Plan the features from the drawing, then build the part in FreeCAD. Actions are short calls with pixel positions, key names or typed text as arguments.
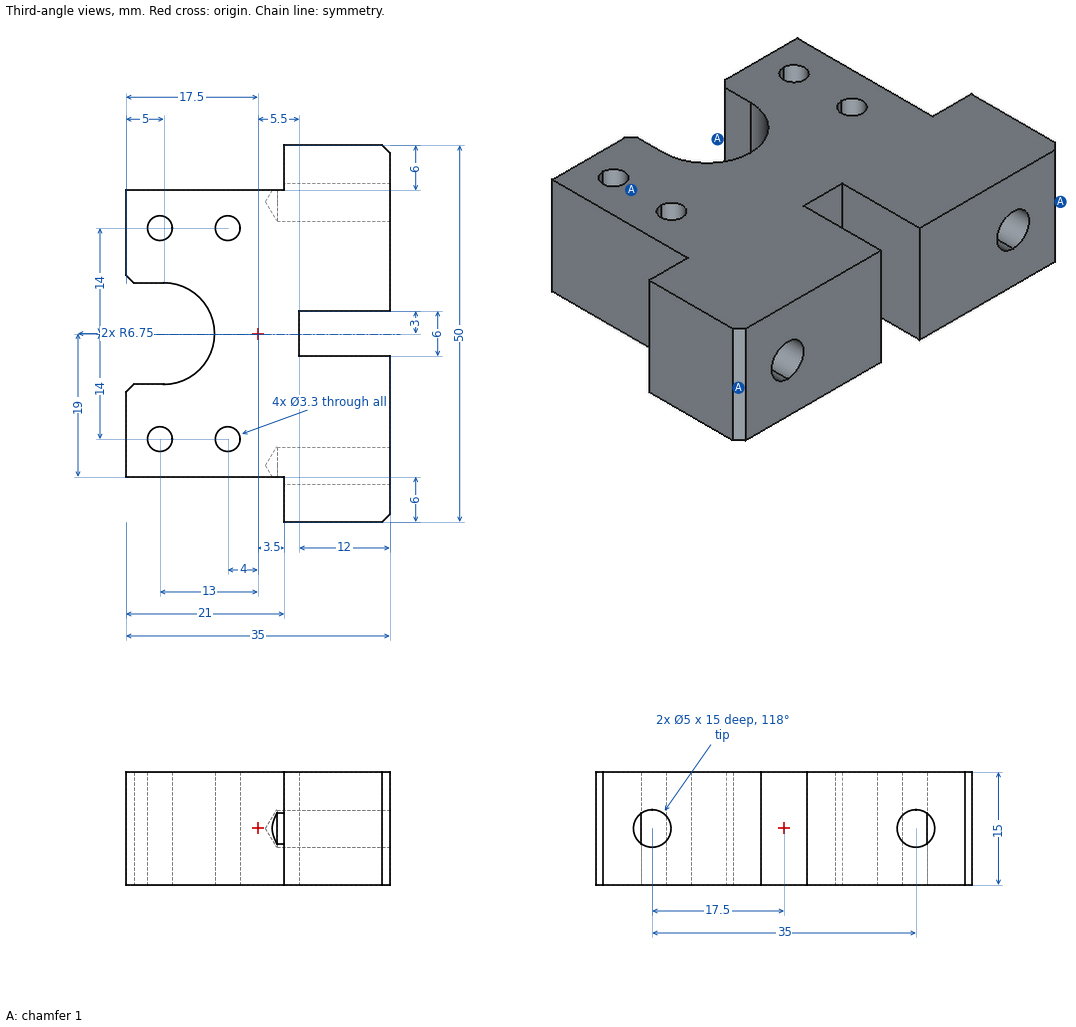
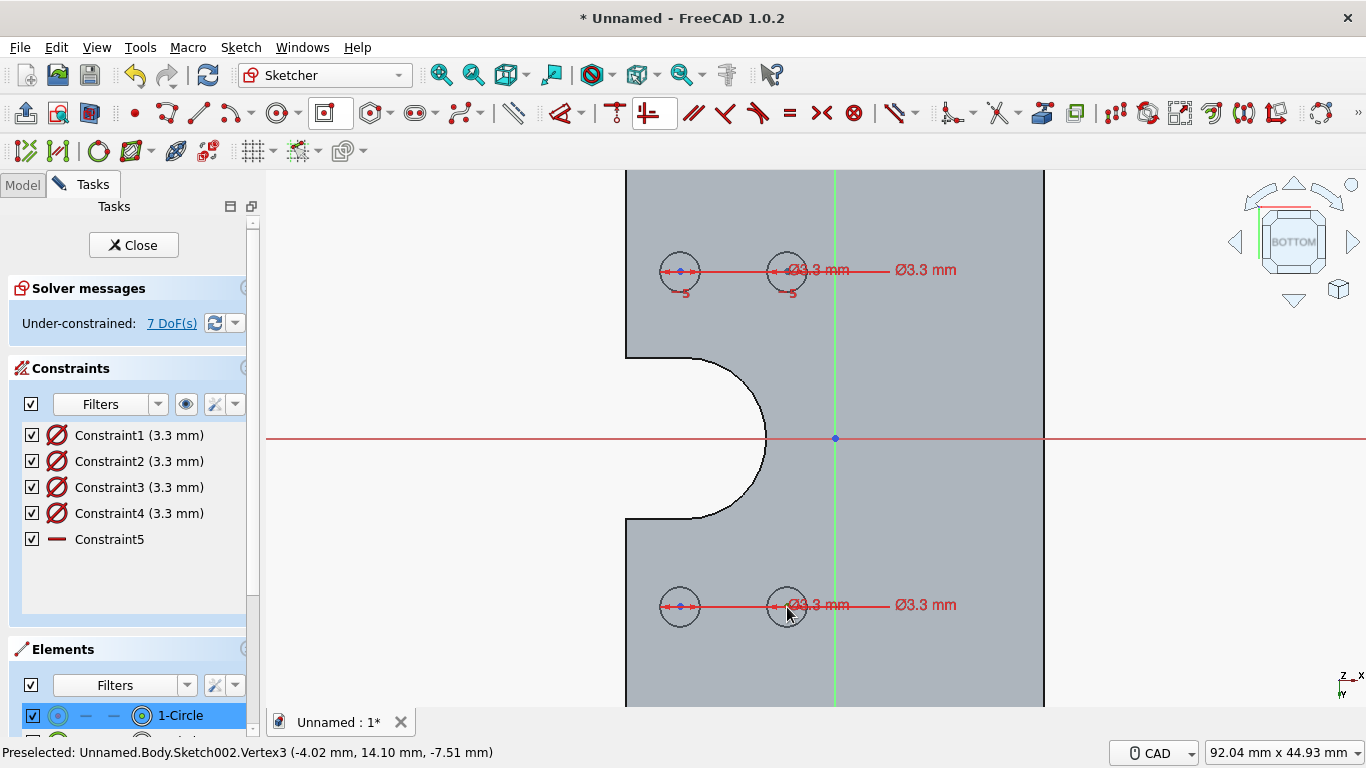
key(v)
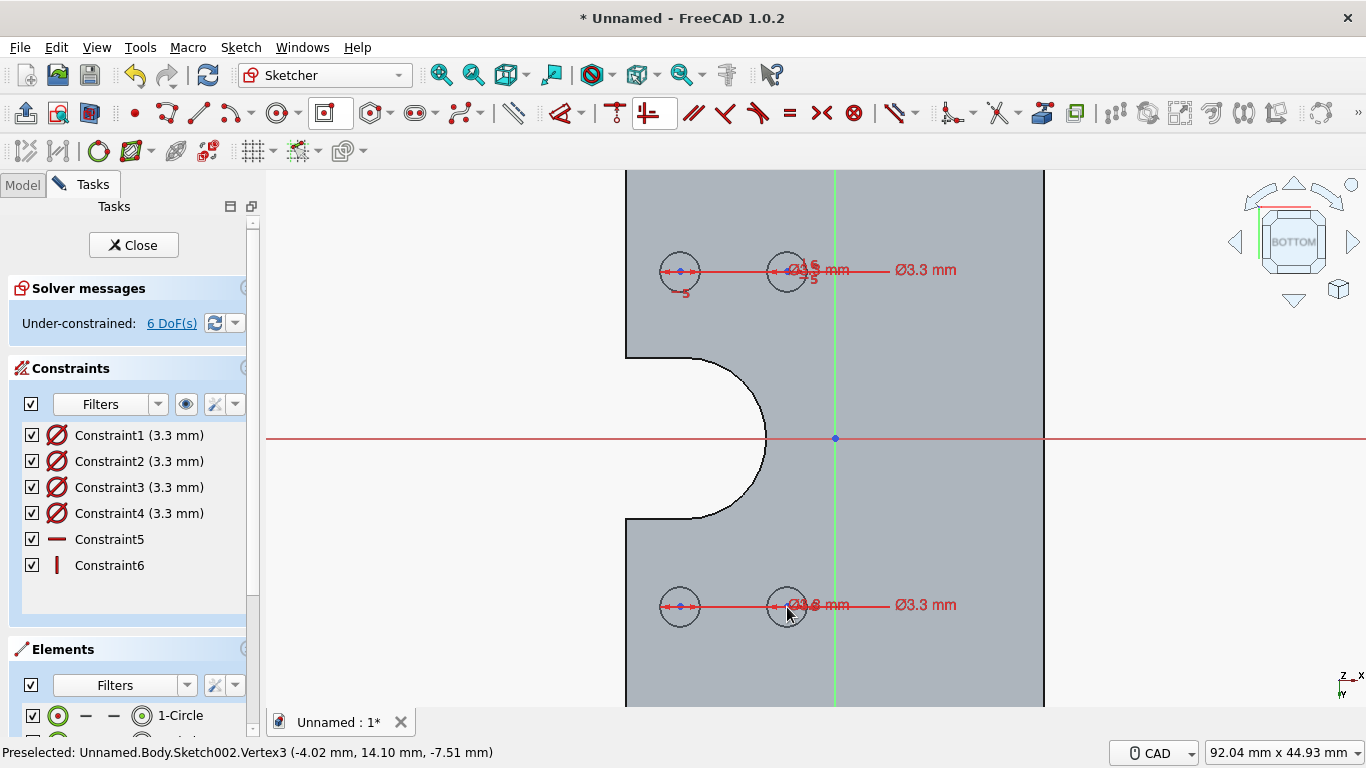
click(680, 272)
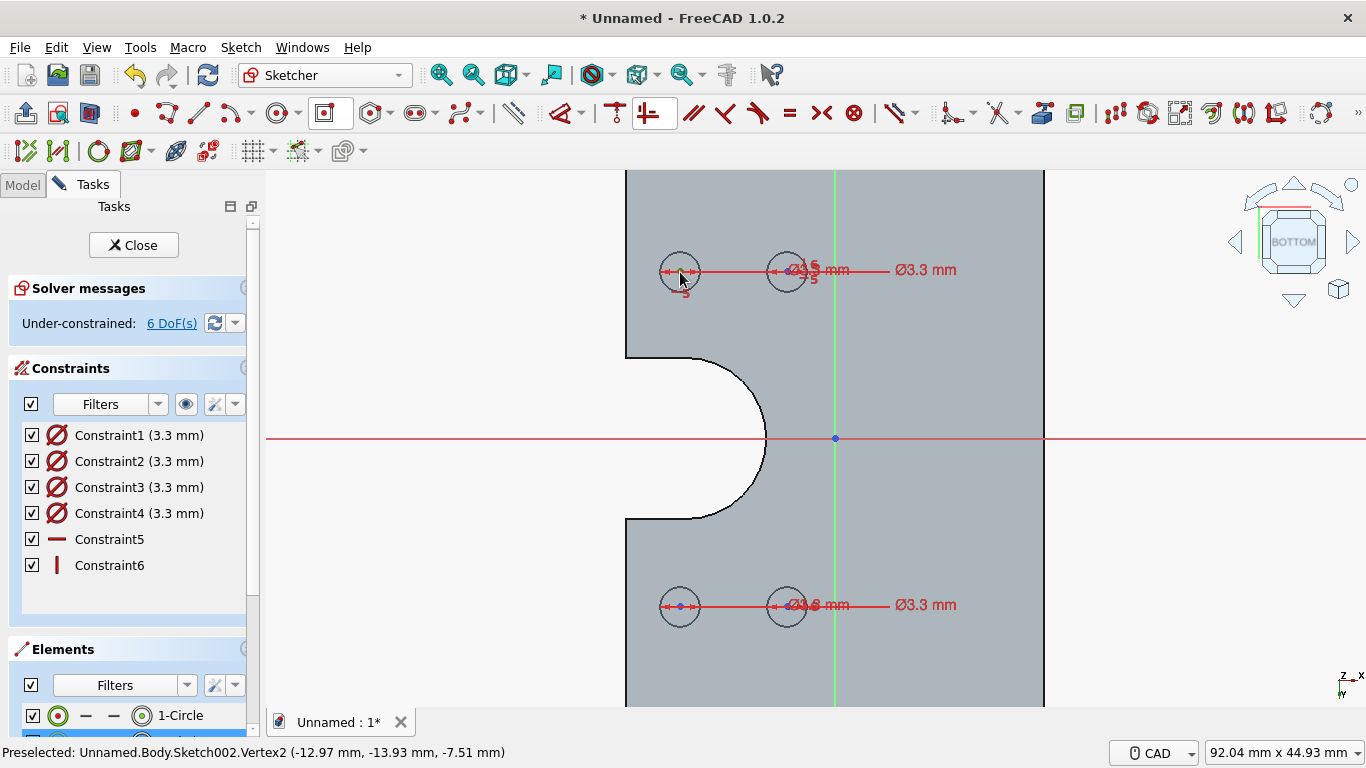
click(680, 607)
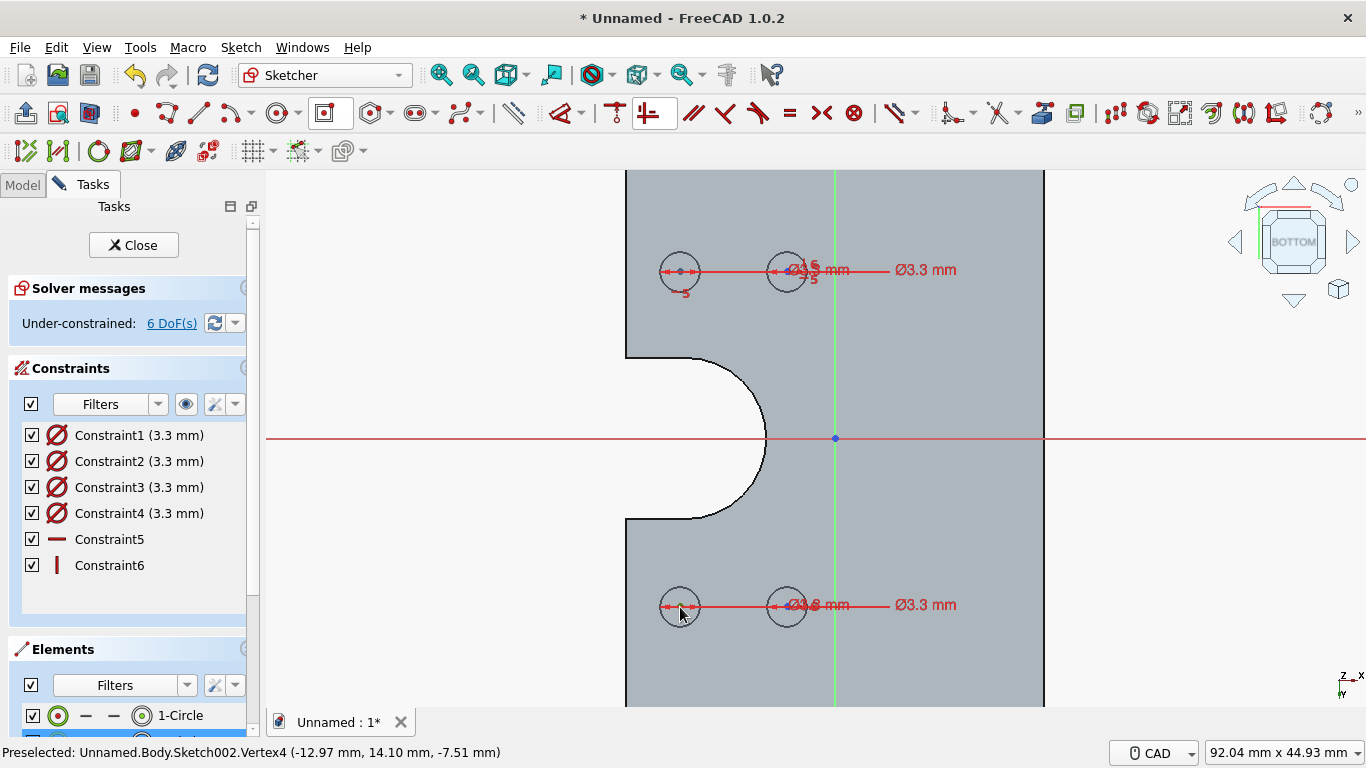
click(672, 114)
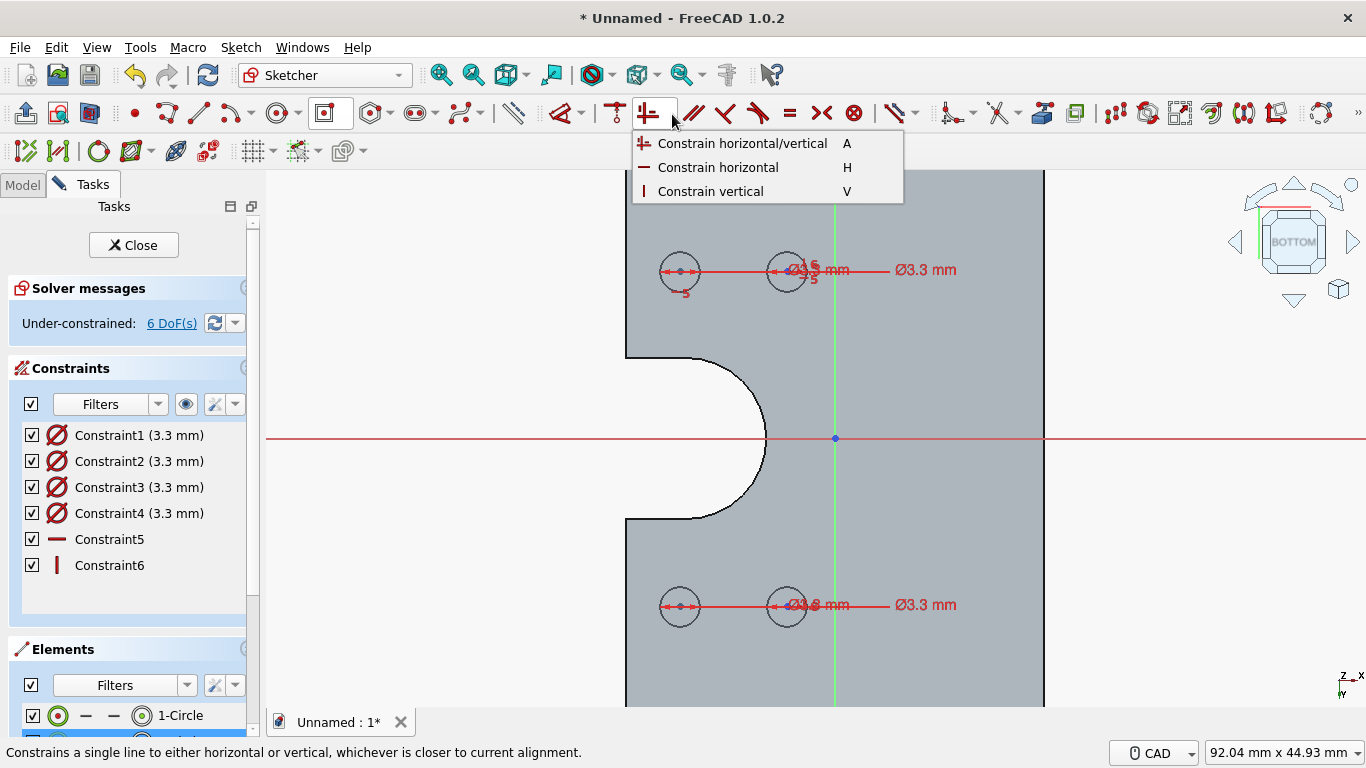
click(768, 191)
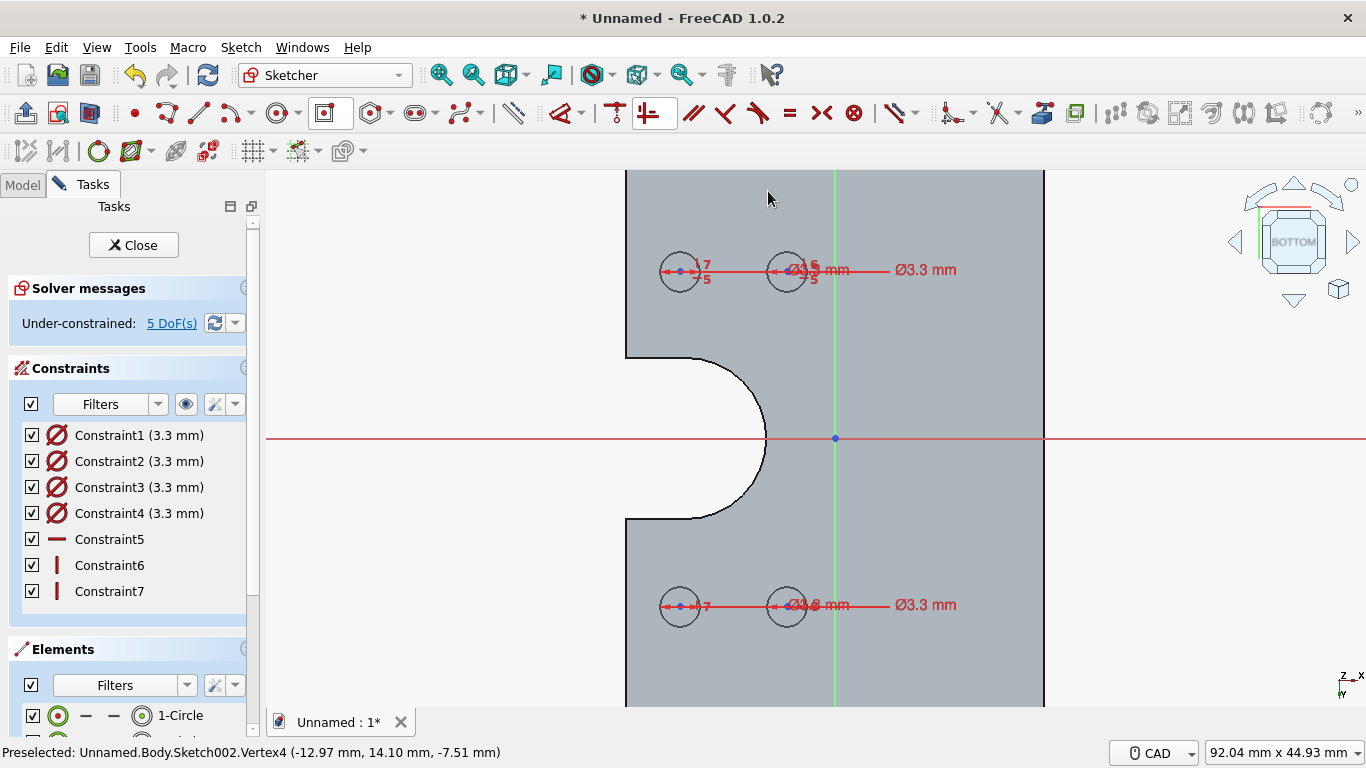
click(787, 607)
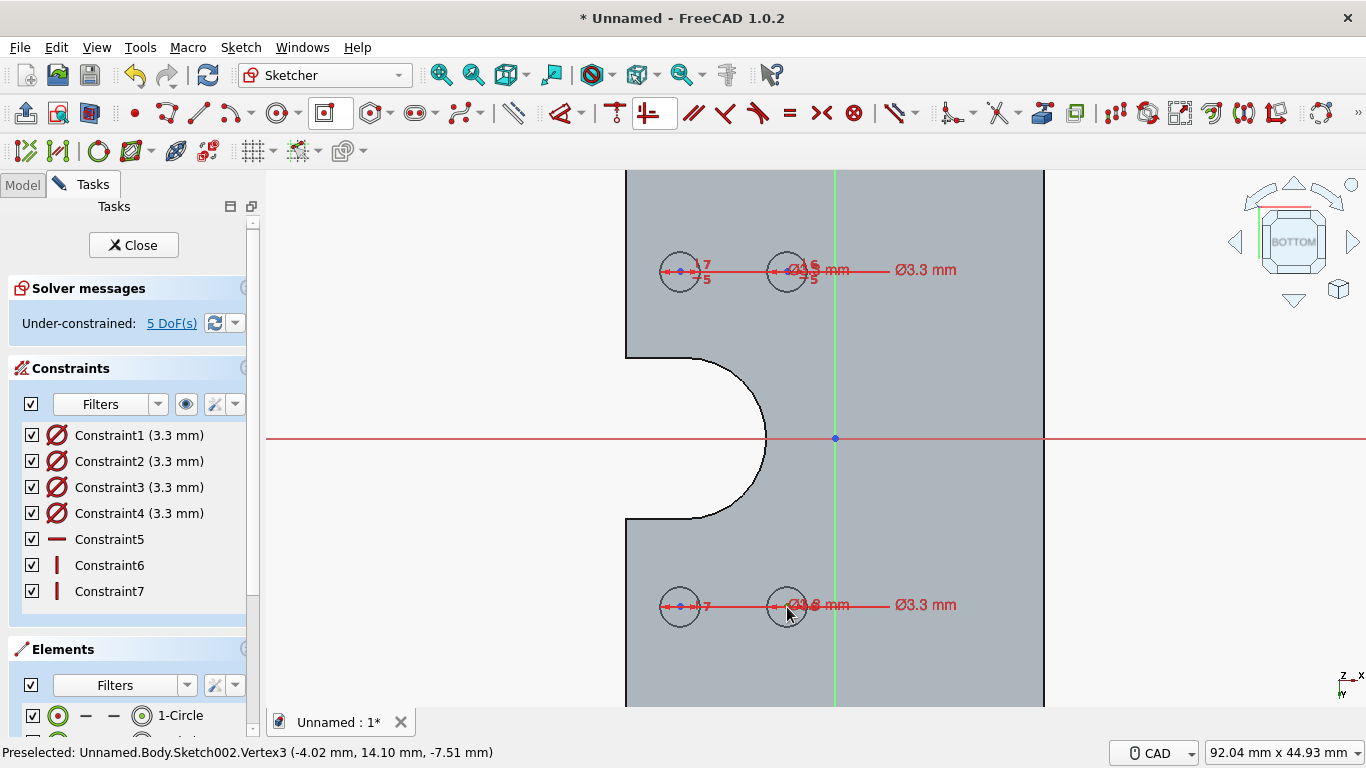
click(680, 607)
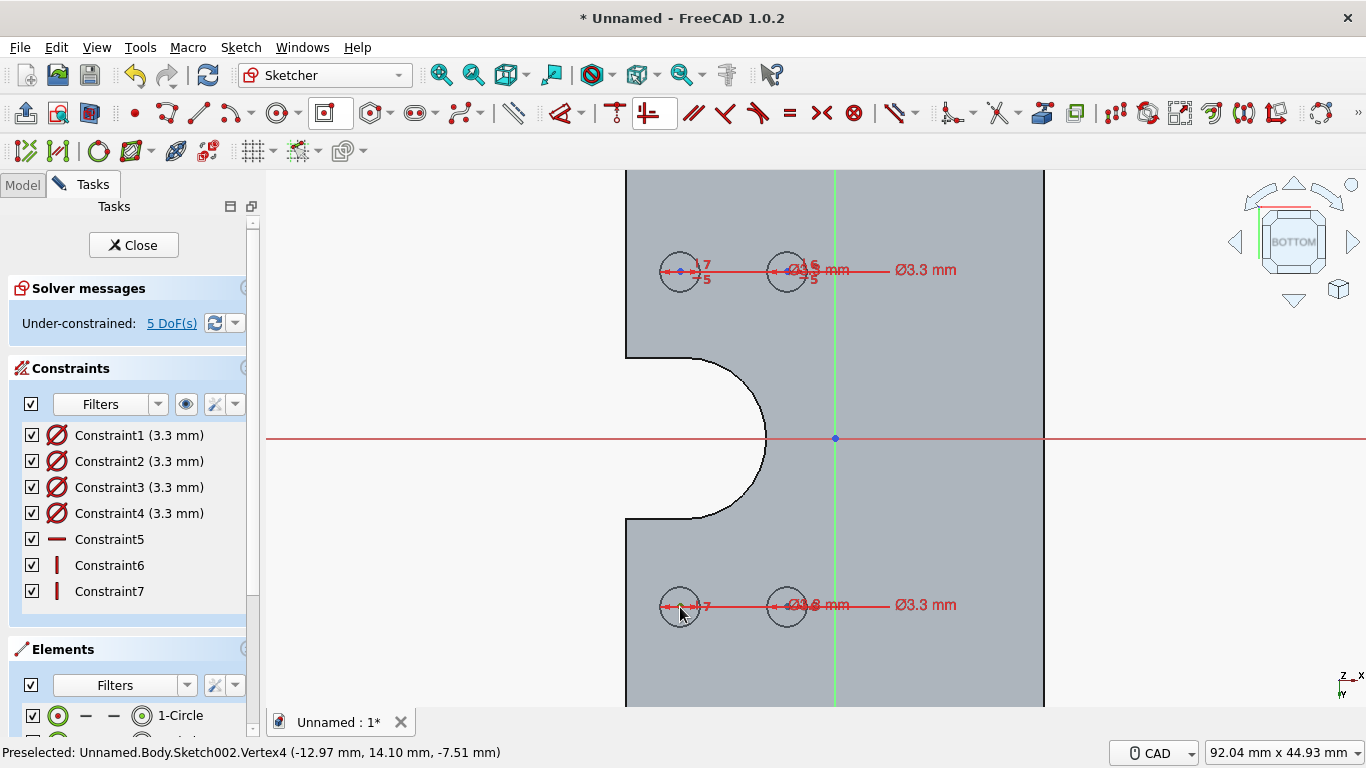
click(672, 114)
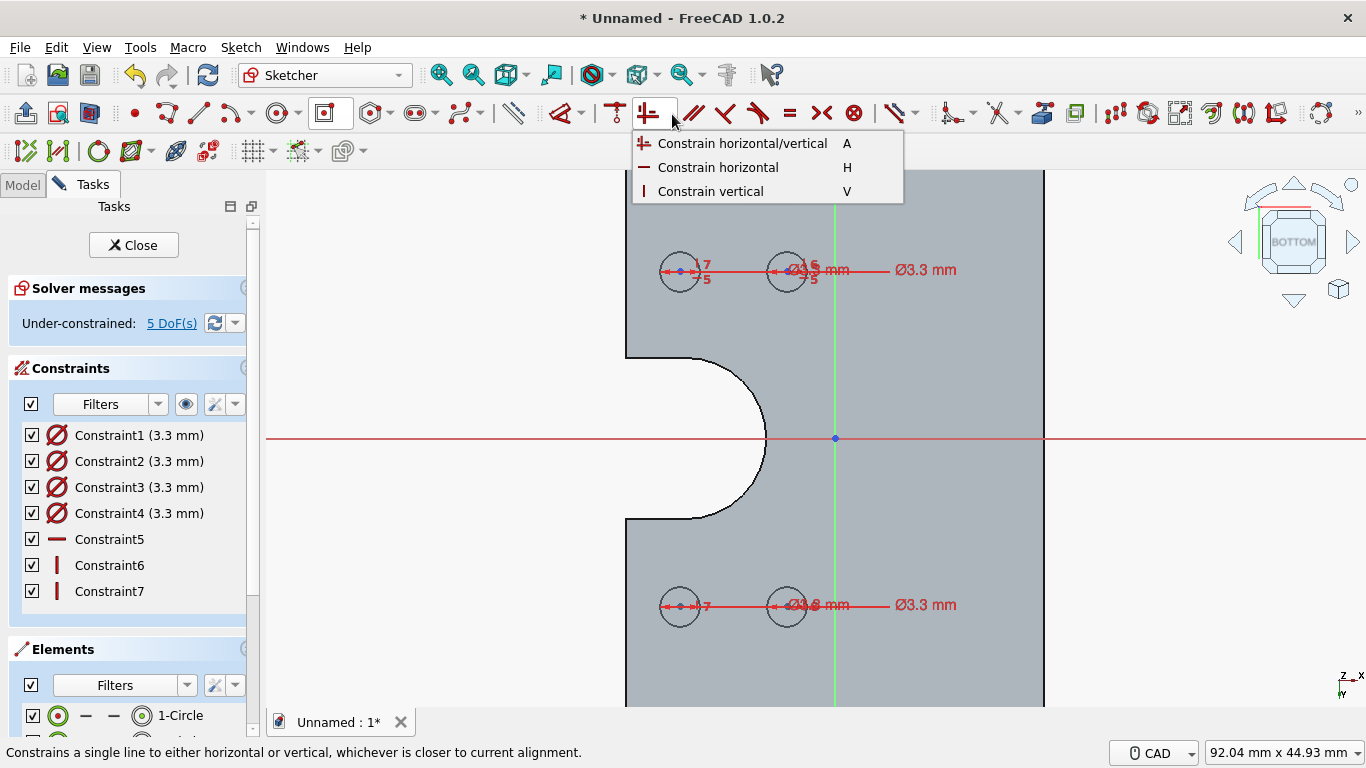
click(768, 167)